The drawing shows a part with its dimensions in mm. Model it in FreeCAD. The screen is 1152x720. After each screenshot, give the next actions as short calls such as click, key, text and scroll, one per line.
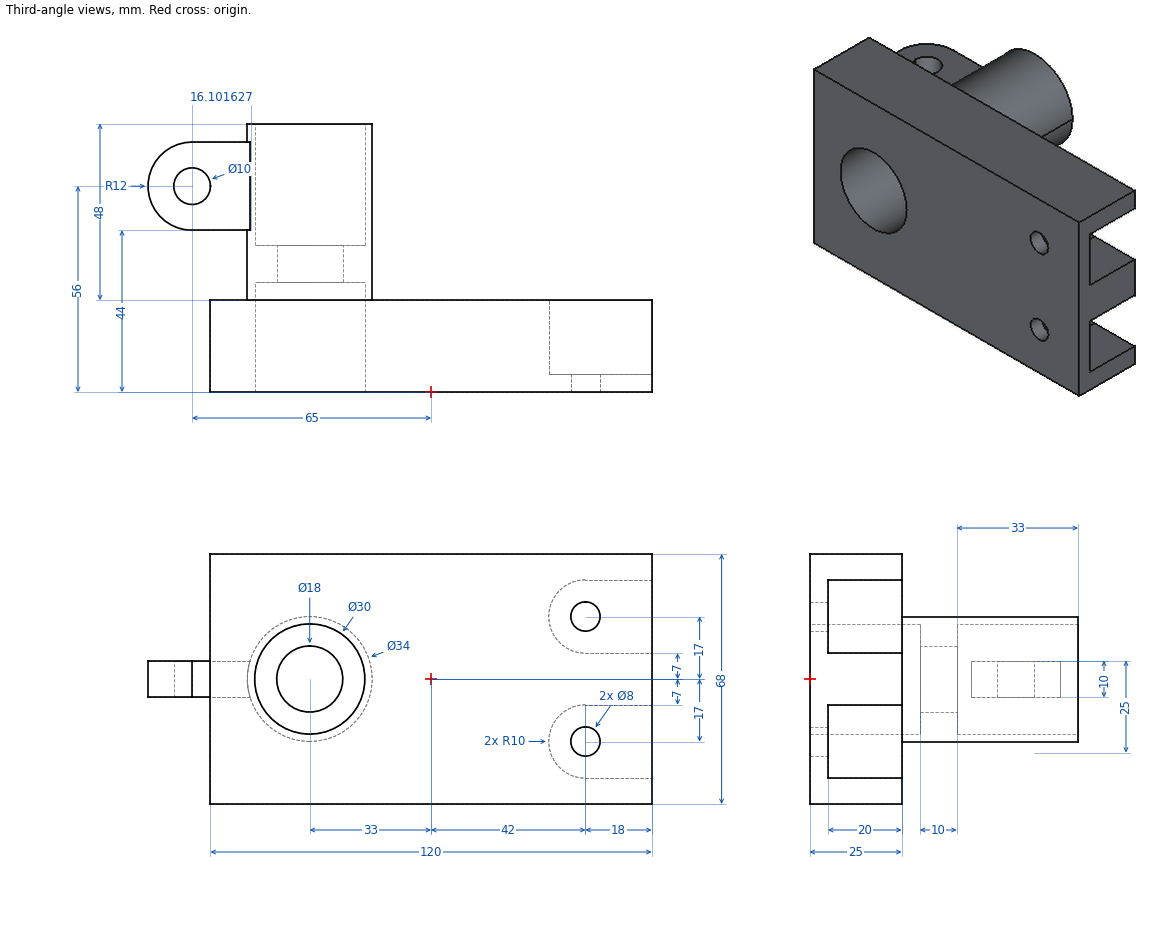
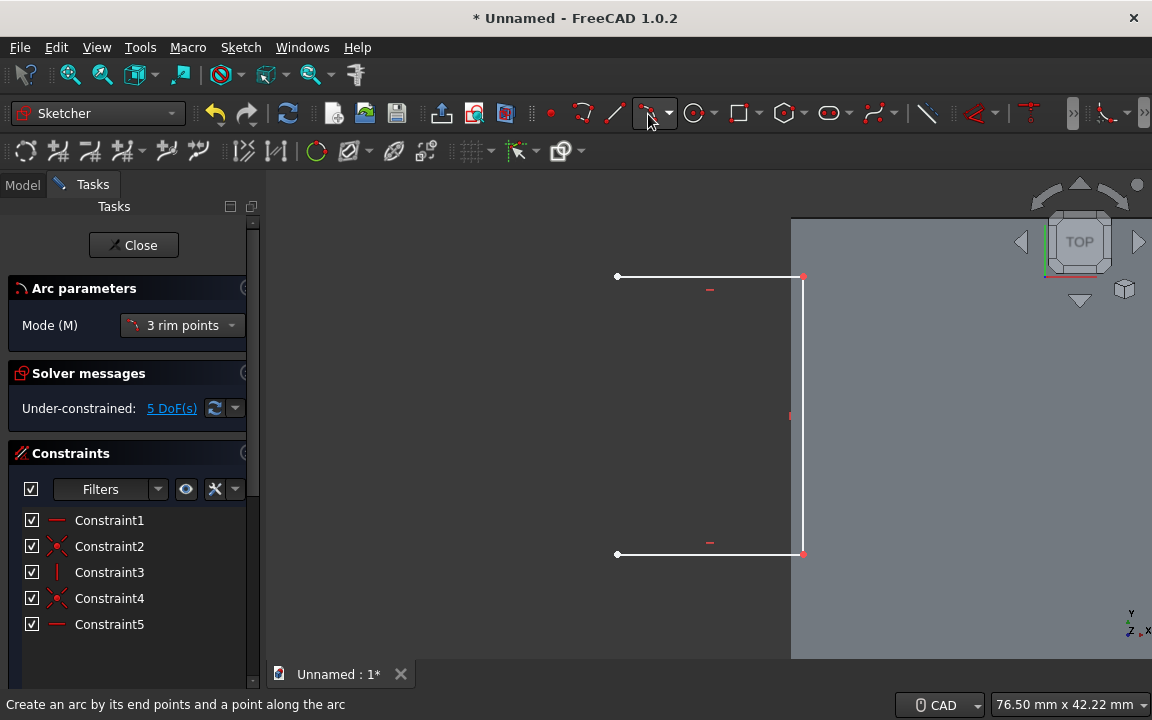
click(617, 277)
click(617, 555)
click(478, 415)
key(Escape)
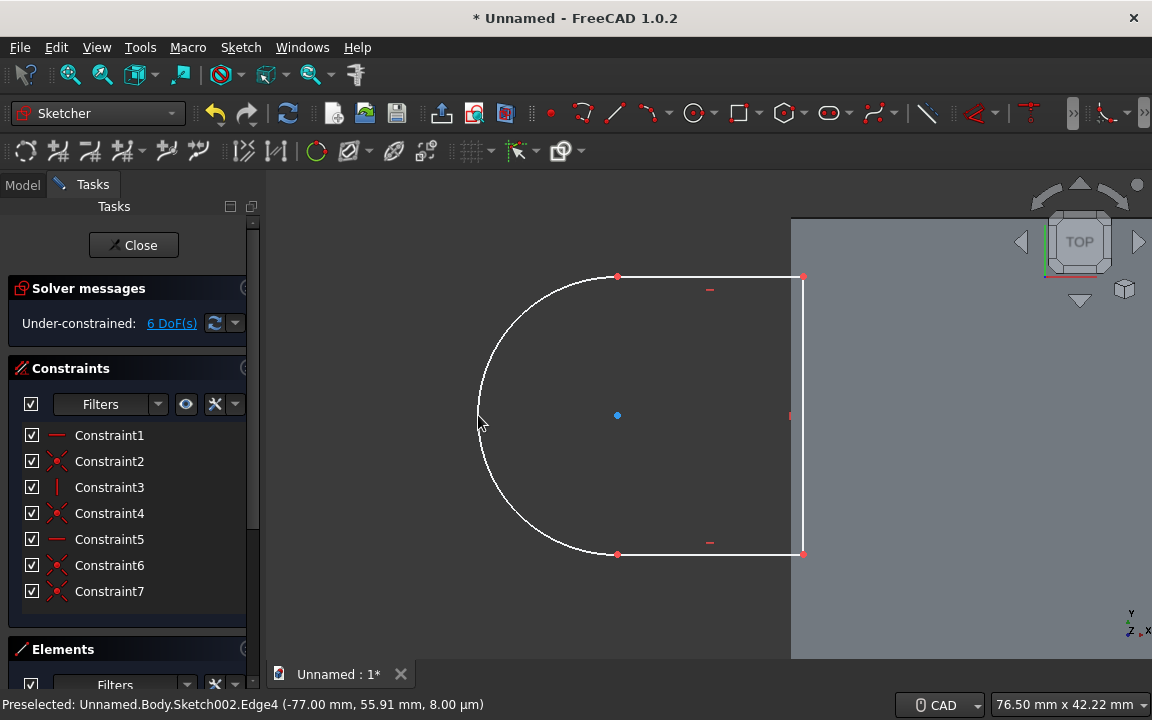
click(673, 555)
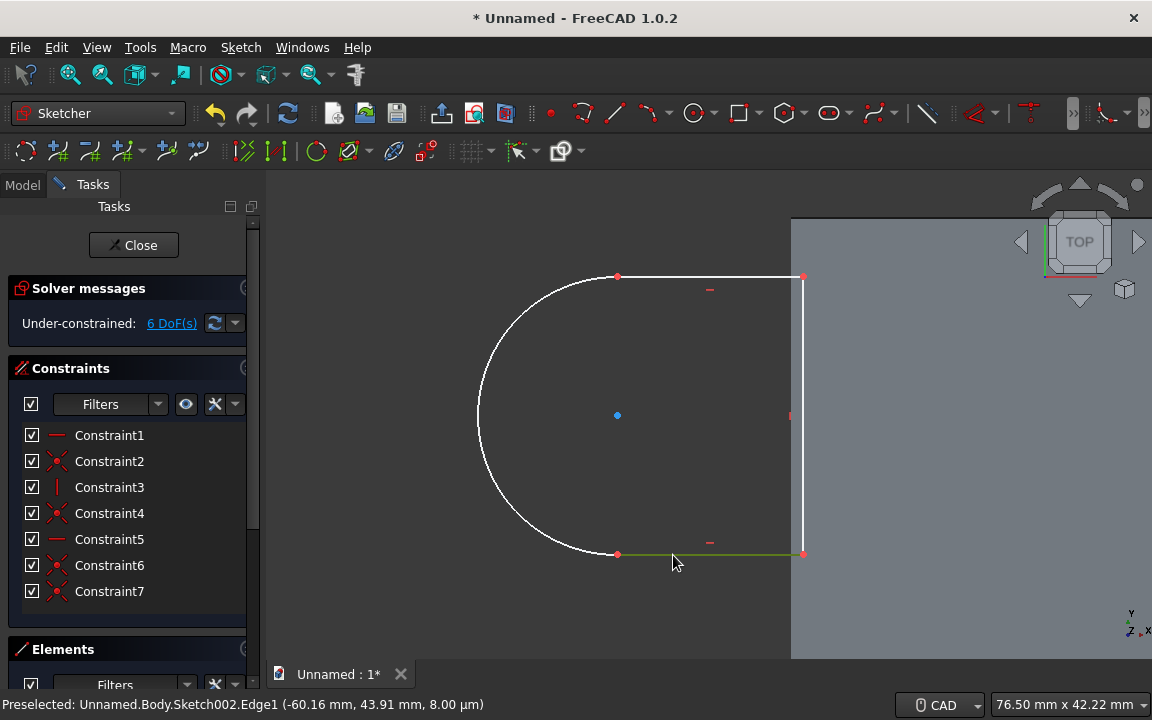
click(505, 334)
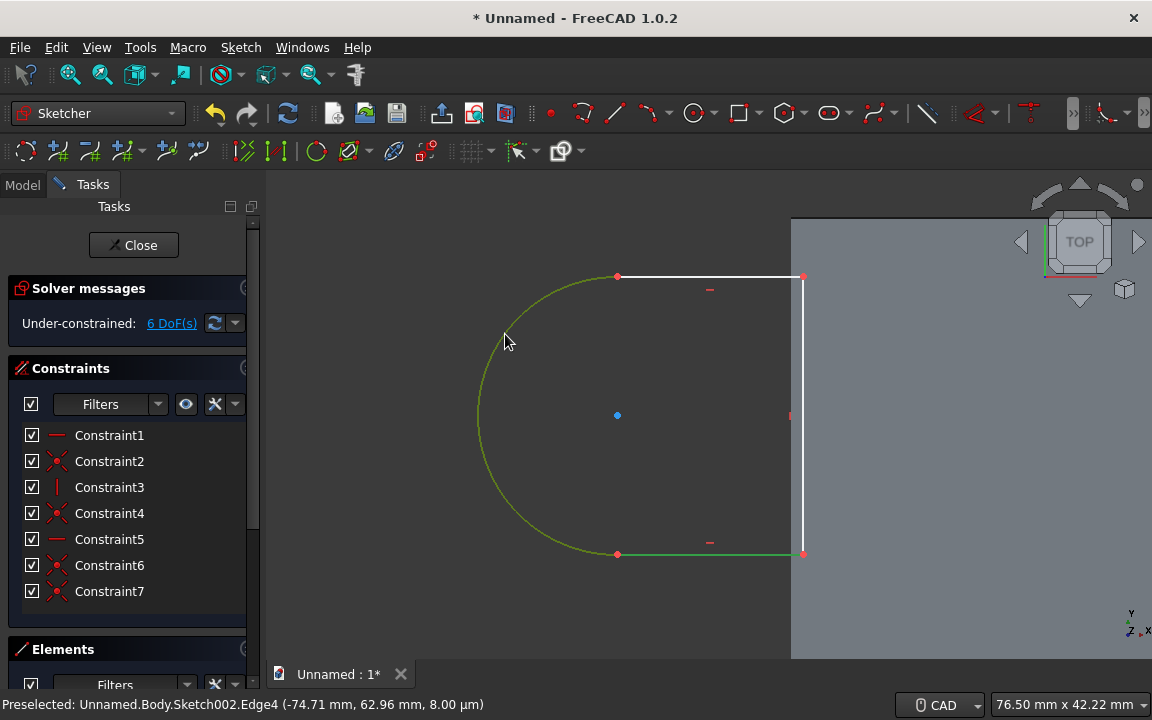
key(t)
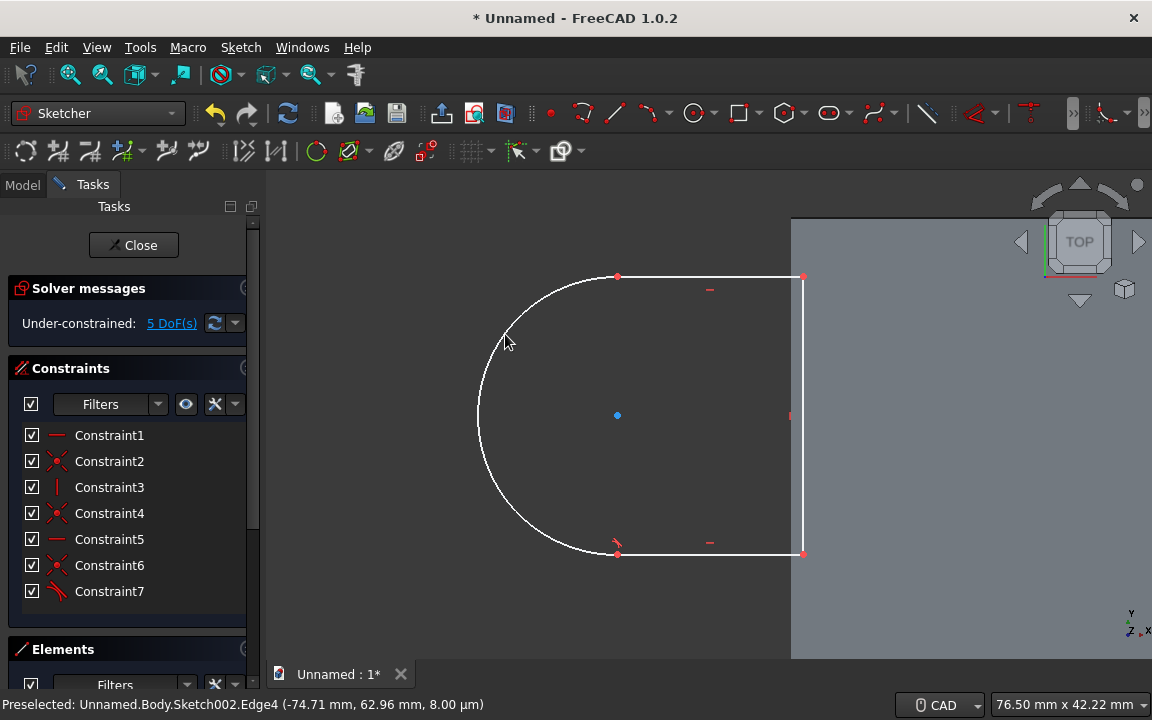
click(747, 277)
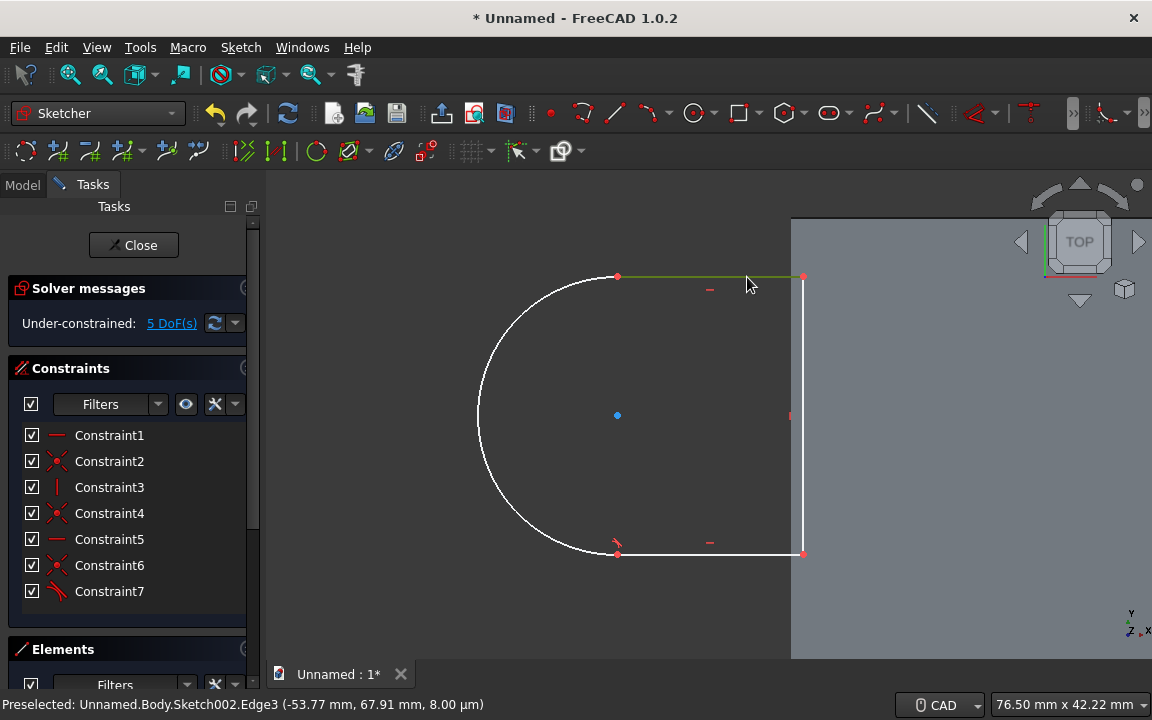
click(505, 334)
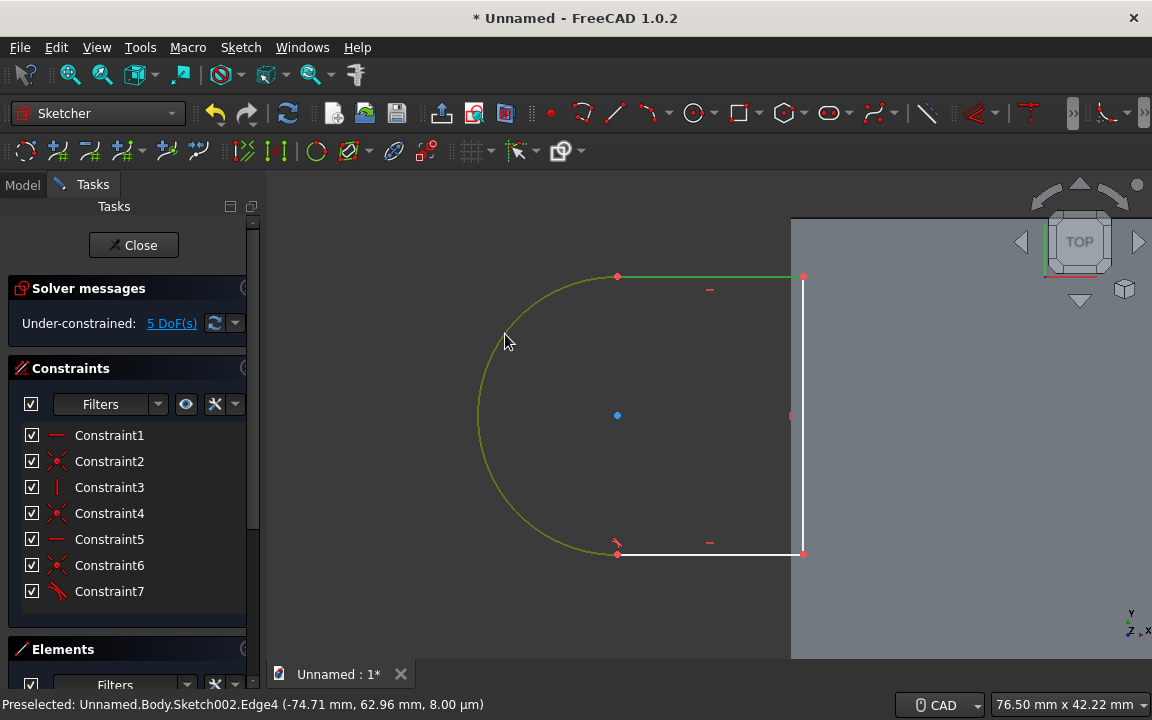
key(t)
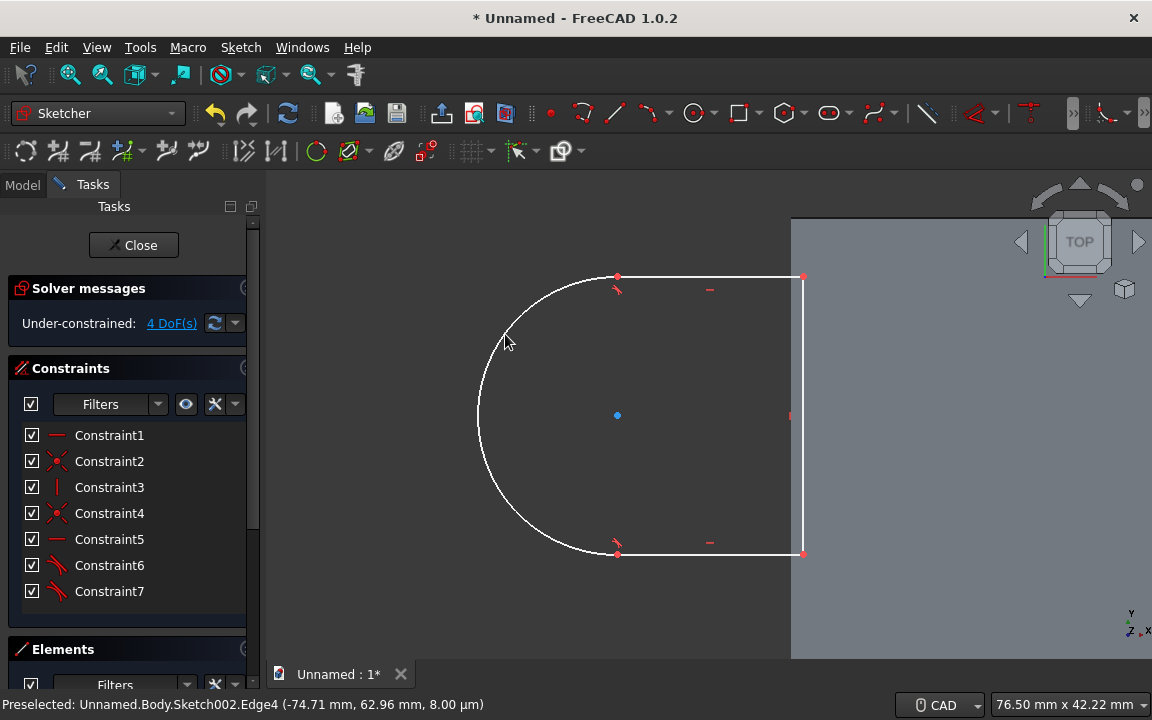
click(974, 114)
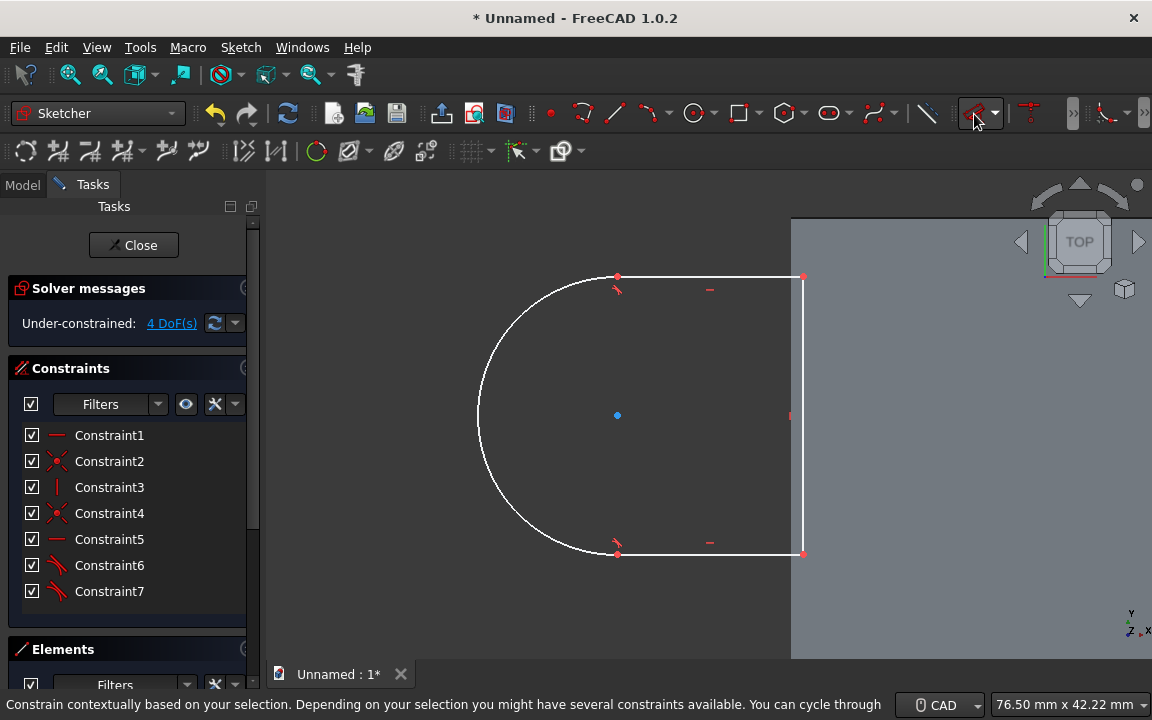
click(505, 334)
click(479, 315)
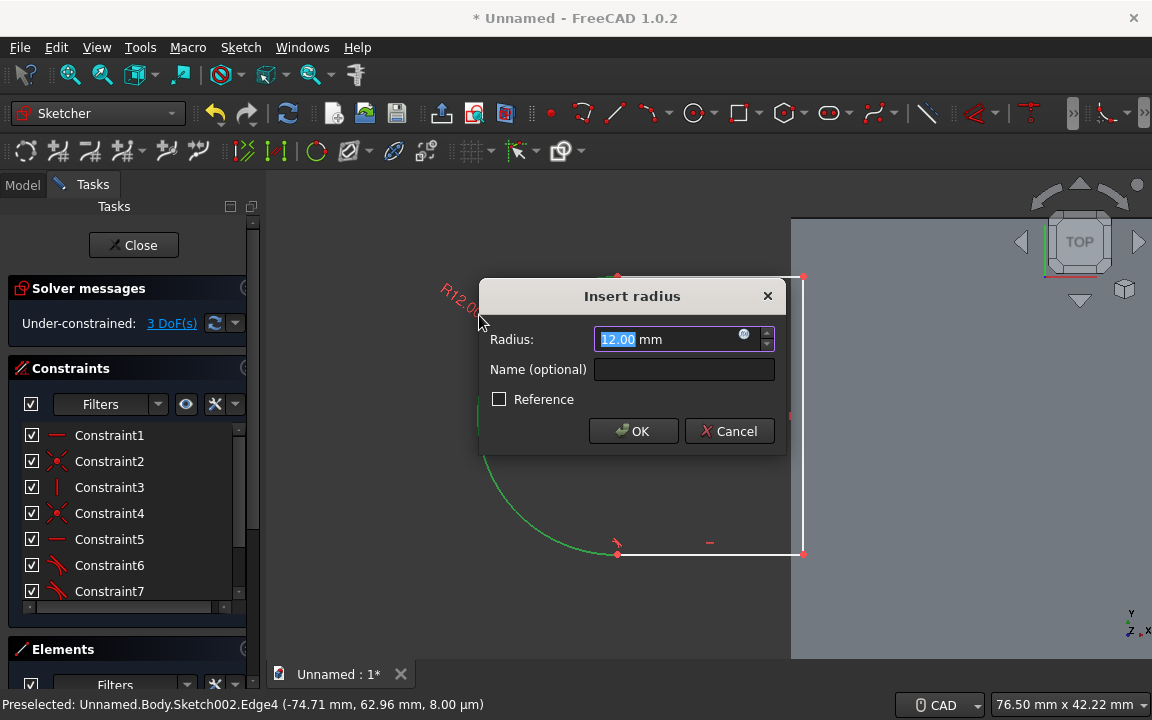
text(12)
key(Return)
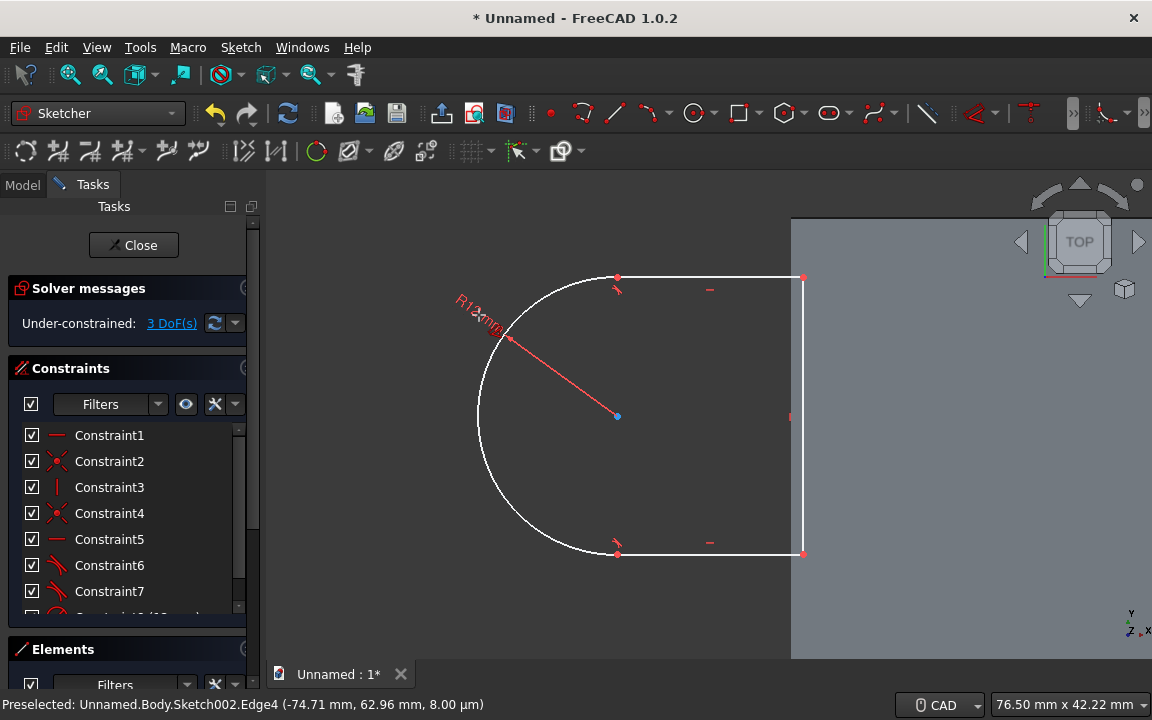
click(617, 555)
click(717, 521)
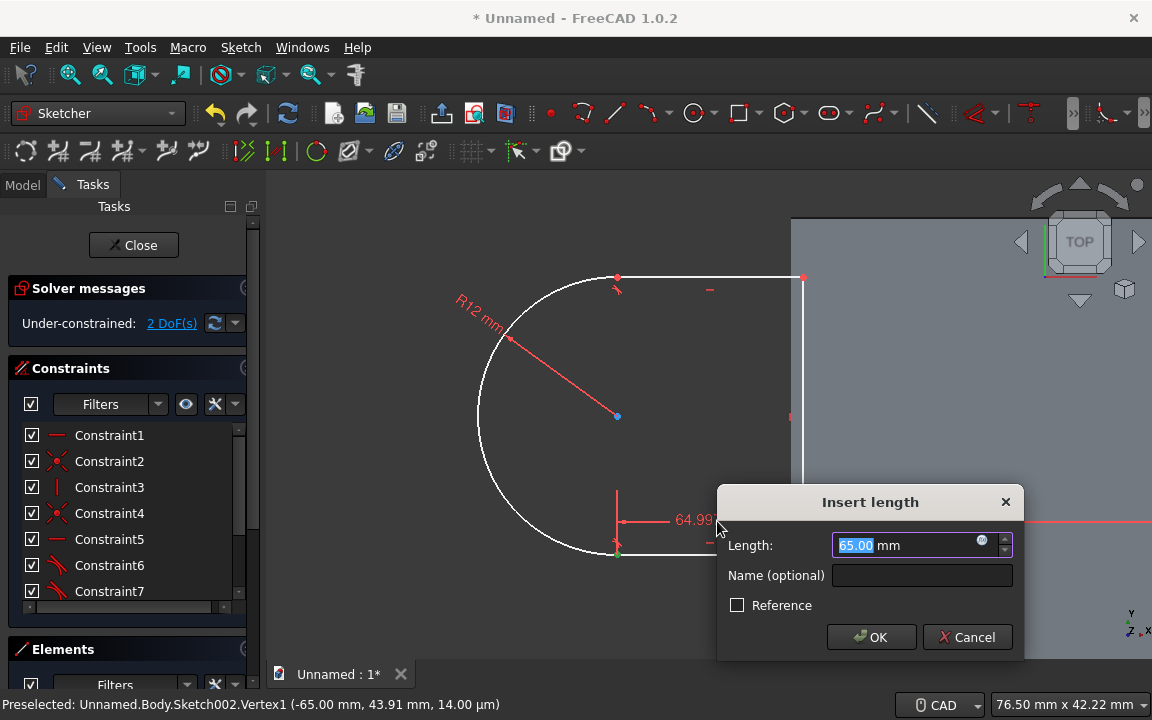
text(65)
key(Return)